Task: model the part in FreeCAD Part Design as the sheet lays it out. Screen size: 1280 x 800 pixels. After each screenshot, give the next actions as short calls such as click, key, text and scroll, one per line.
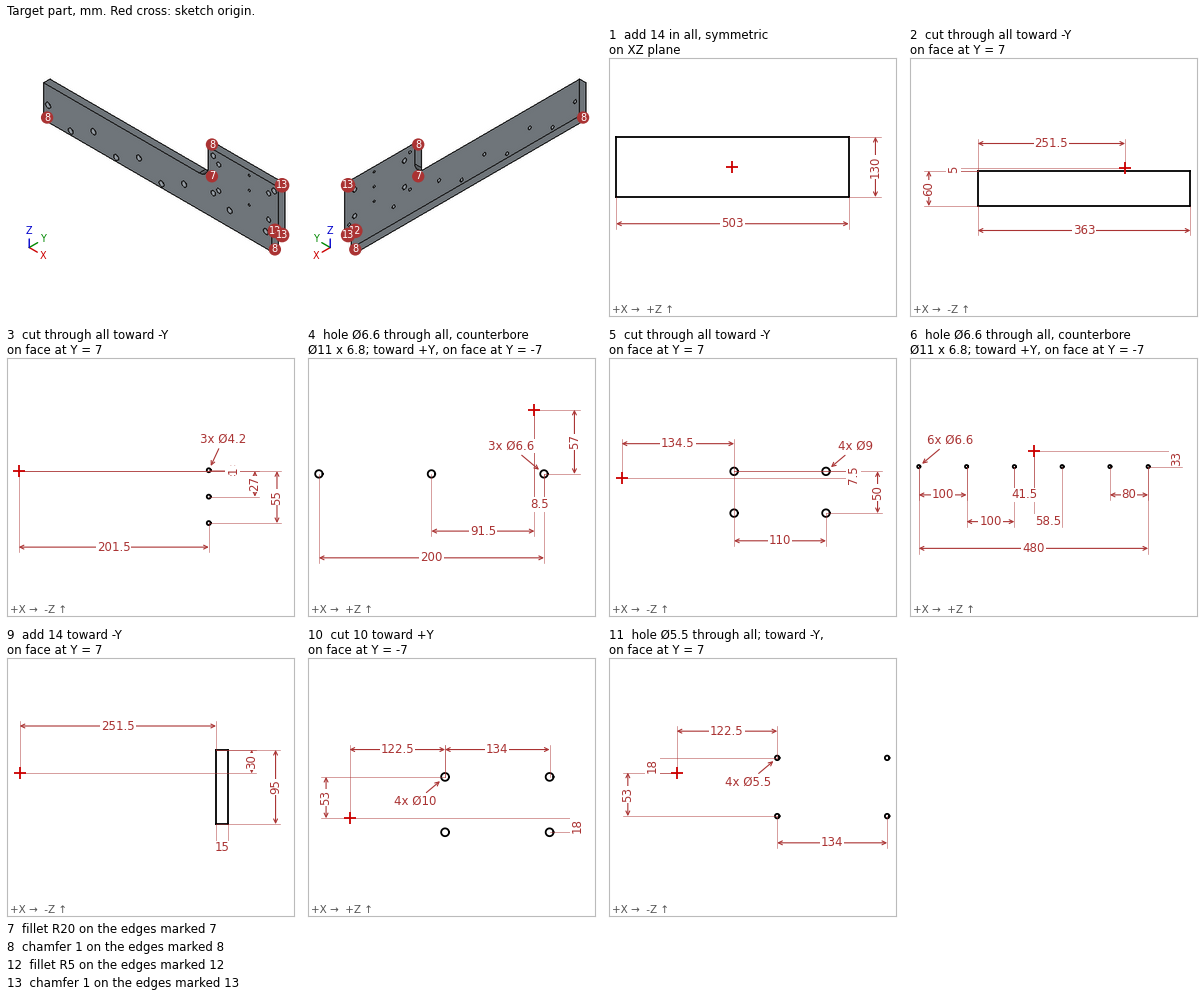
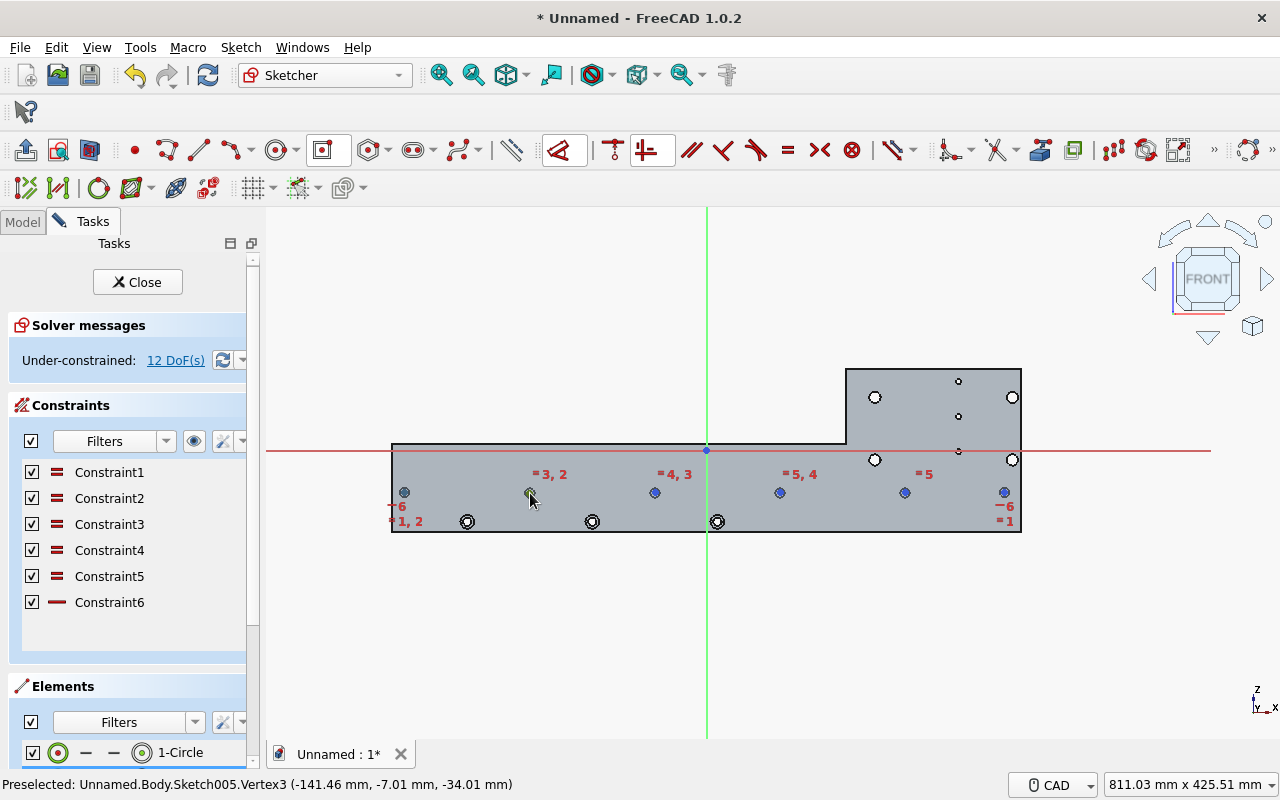
key(h)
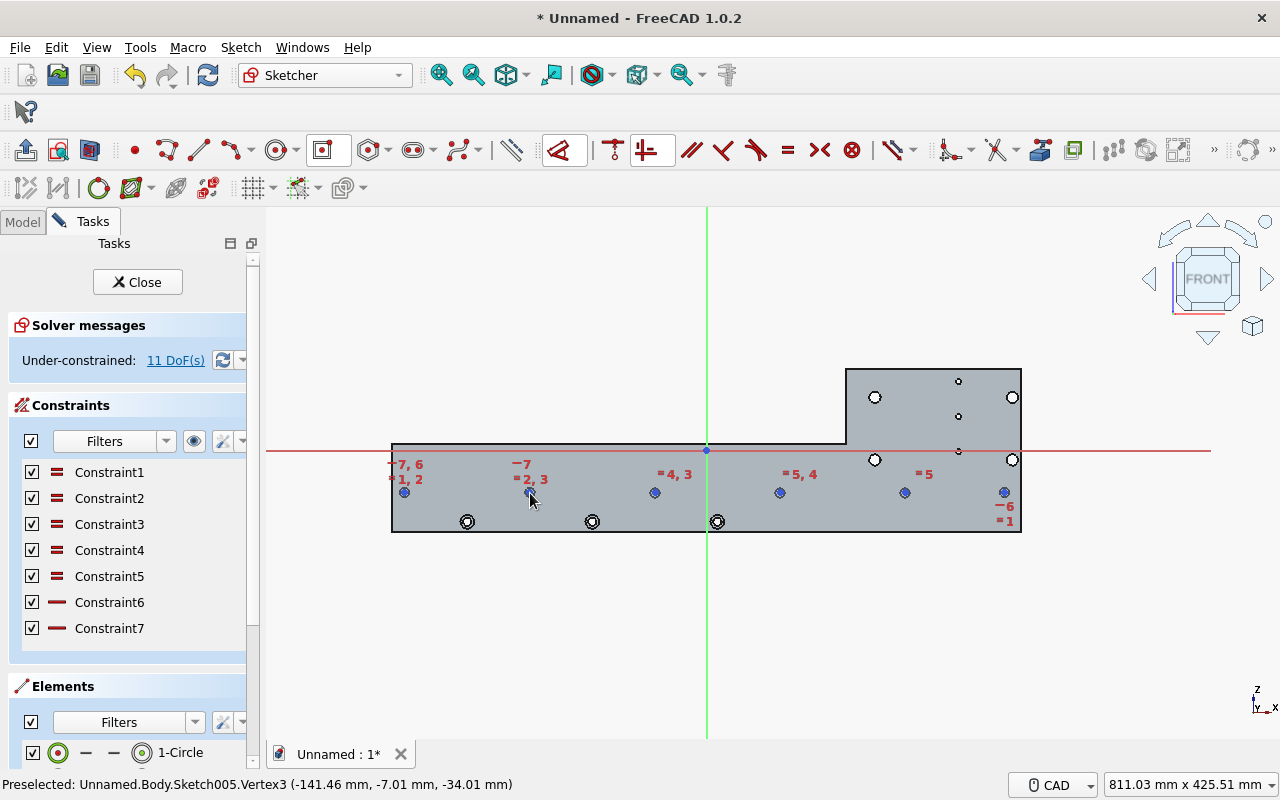
click(530, 492)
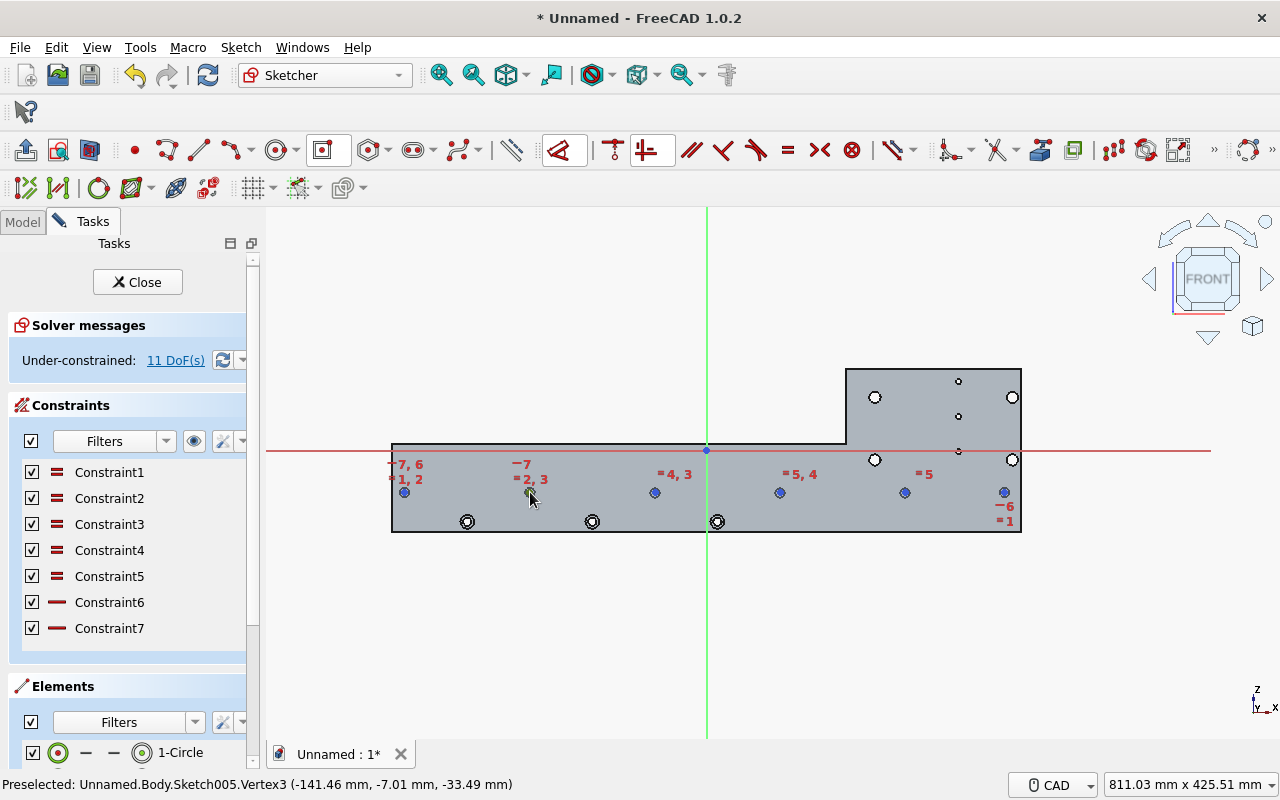
click(655, 493)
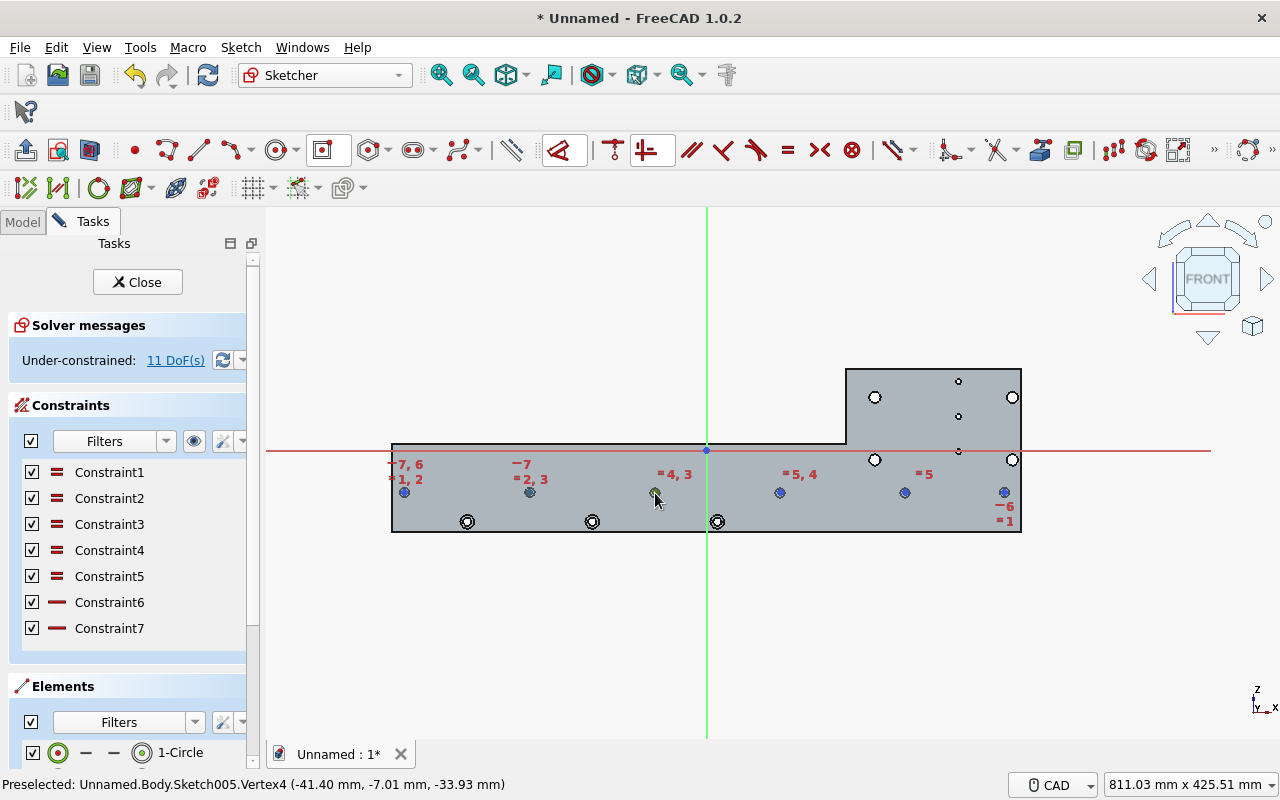
click(670, 150)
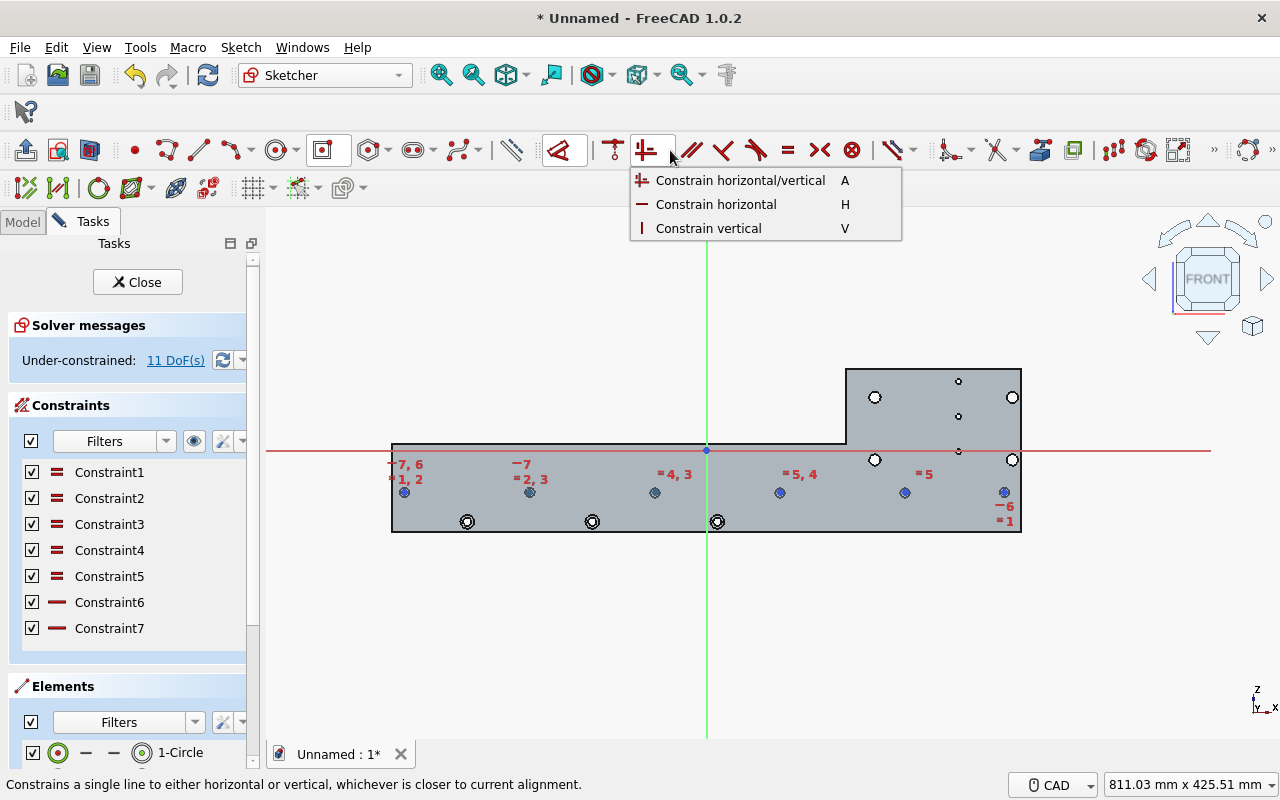
click(766, 204)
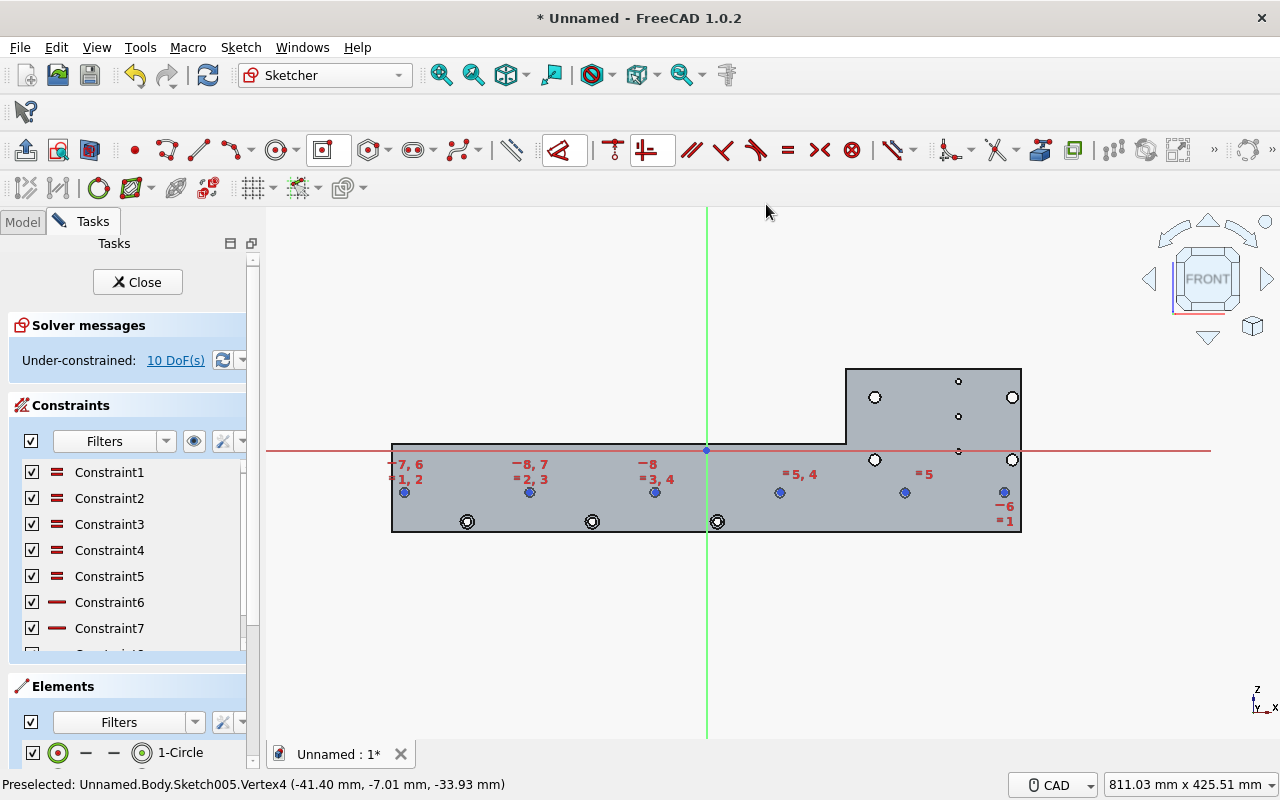
click(655, 492)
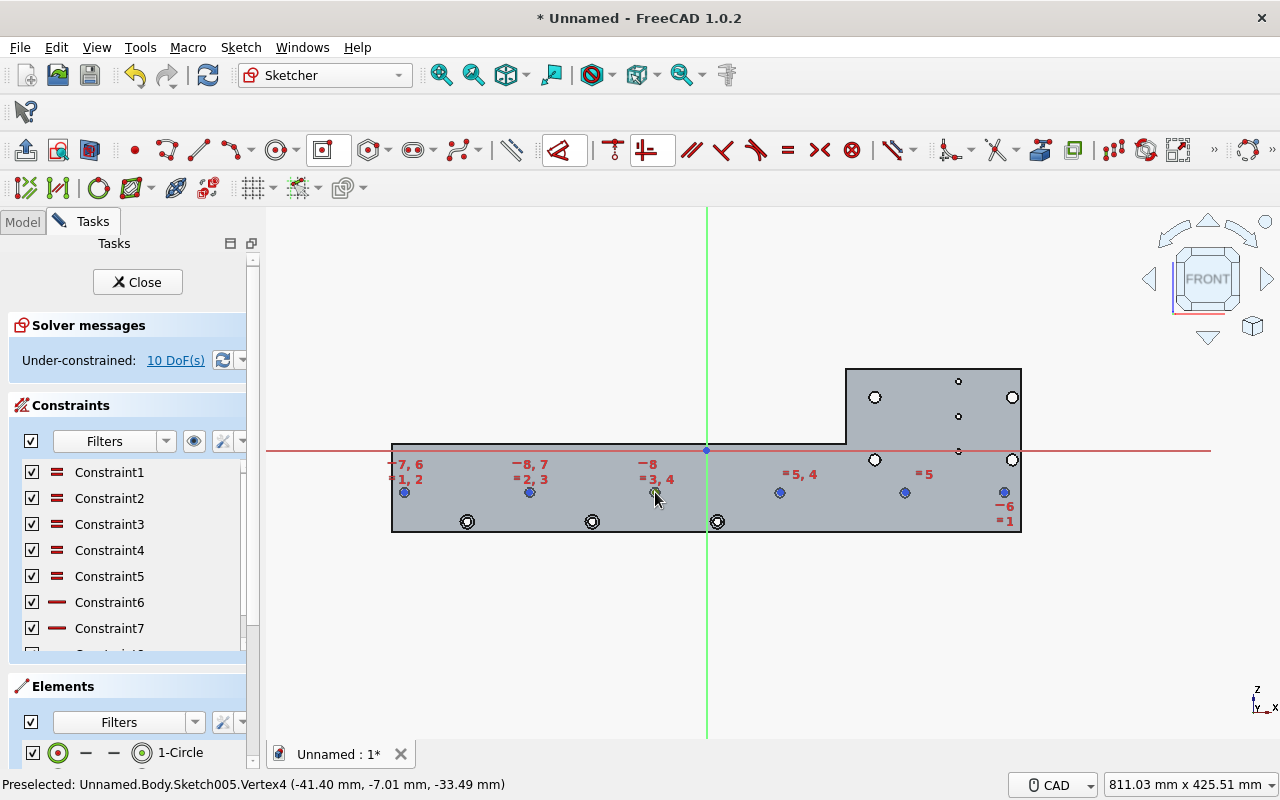
click(780, 493)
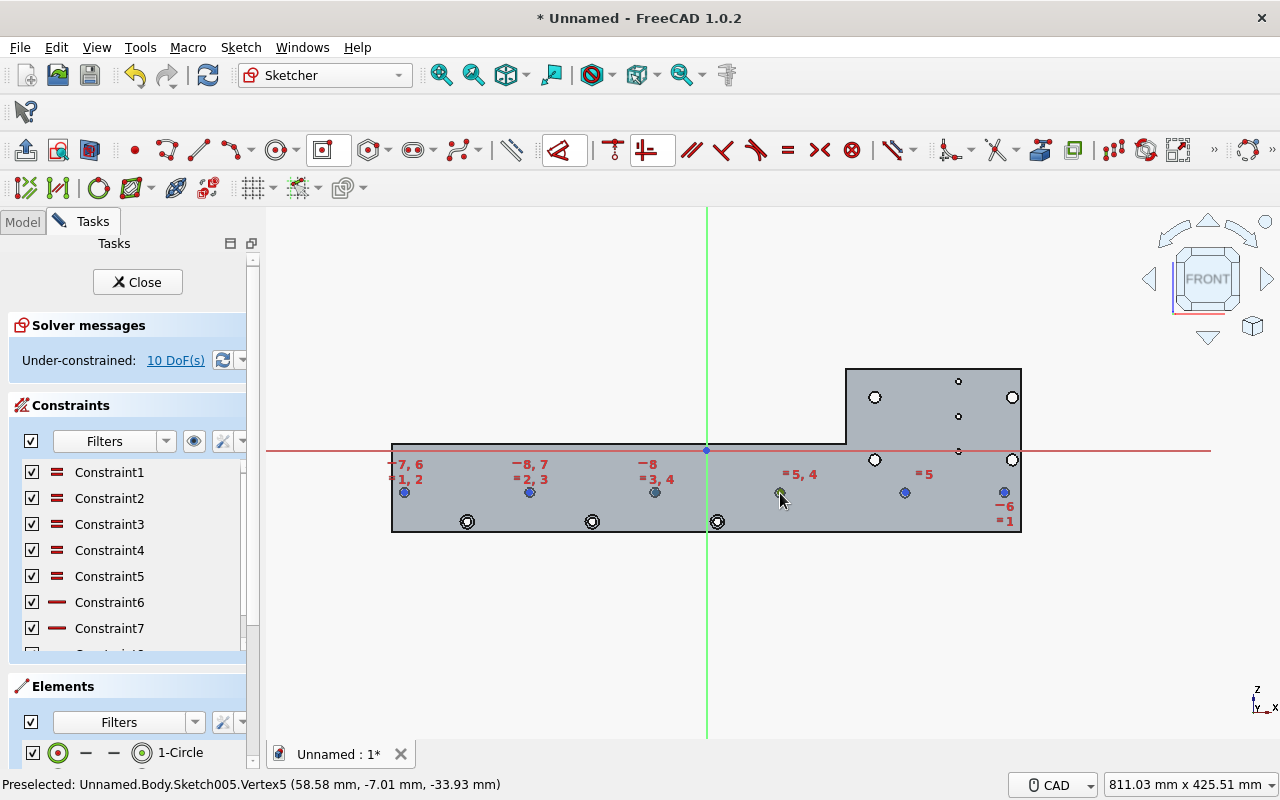
key(h)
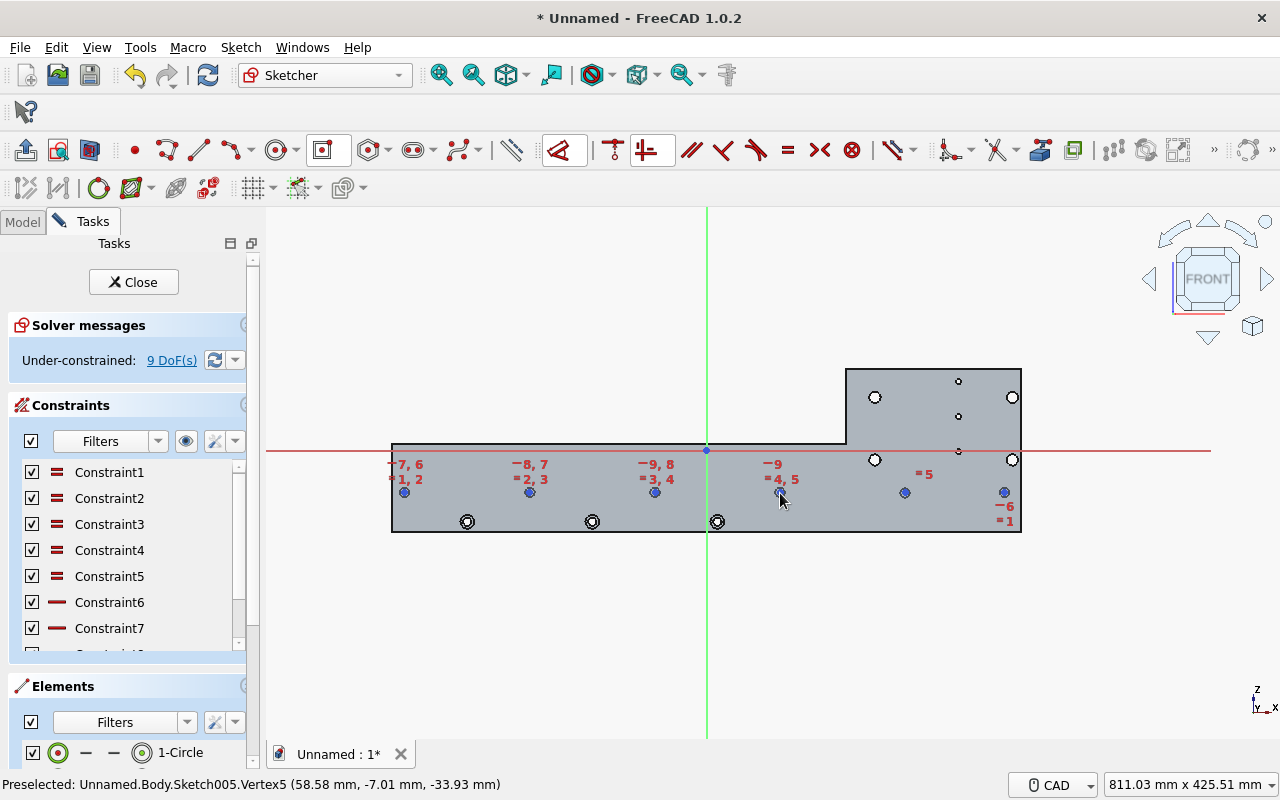
click(1005, 492)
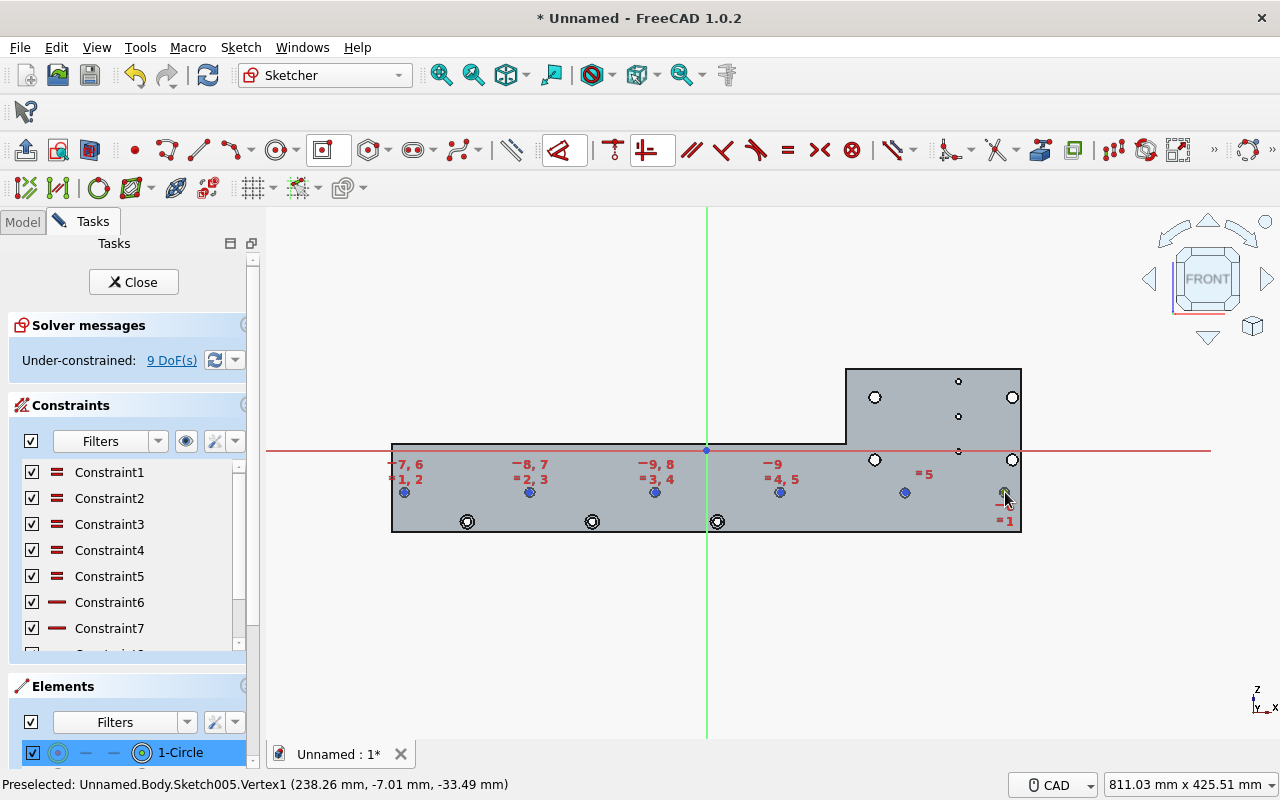
click(905, 493)